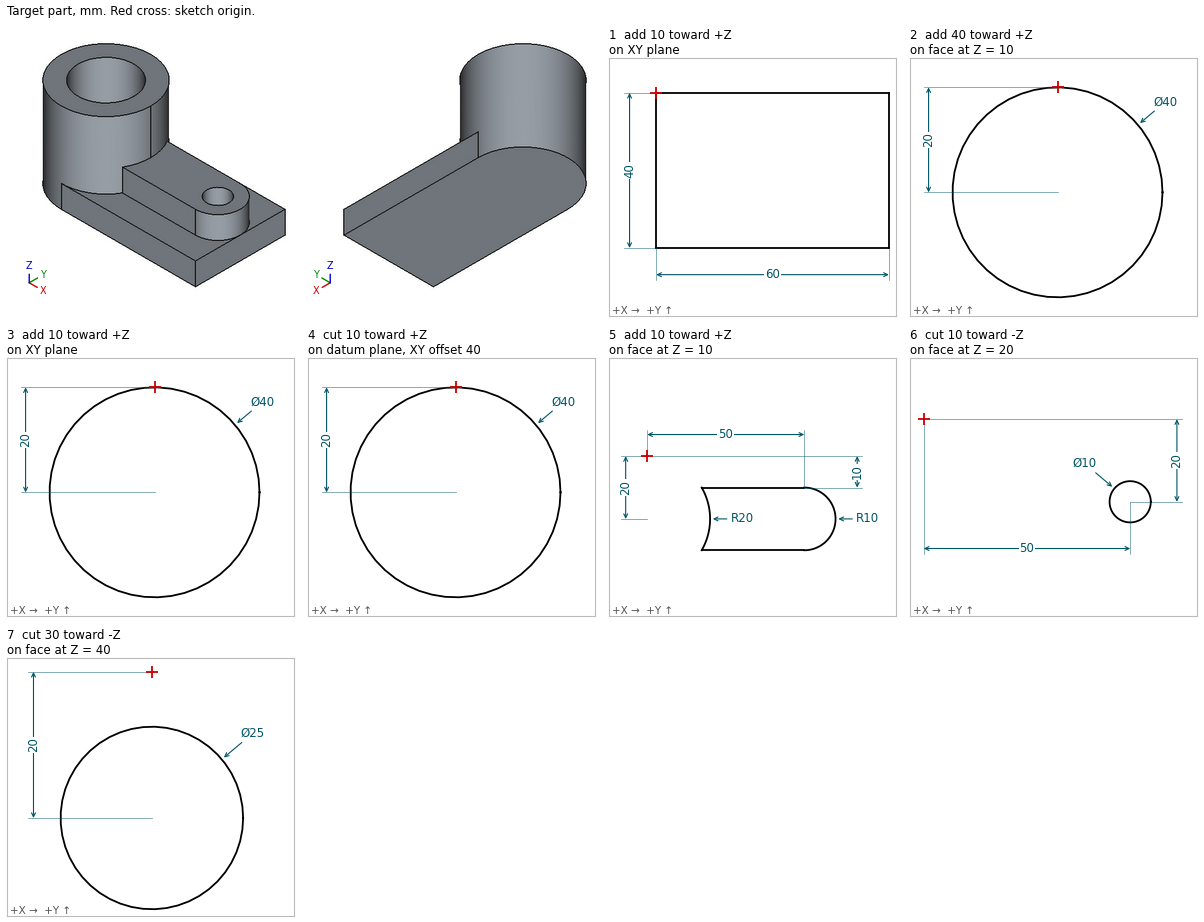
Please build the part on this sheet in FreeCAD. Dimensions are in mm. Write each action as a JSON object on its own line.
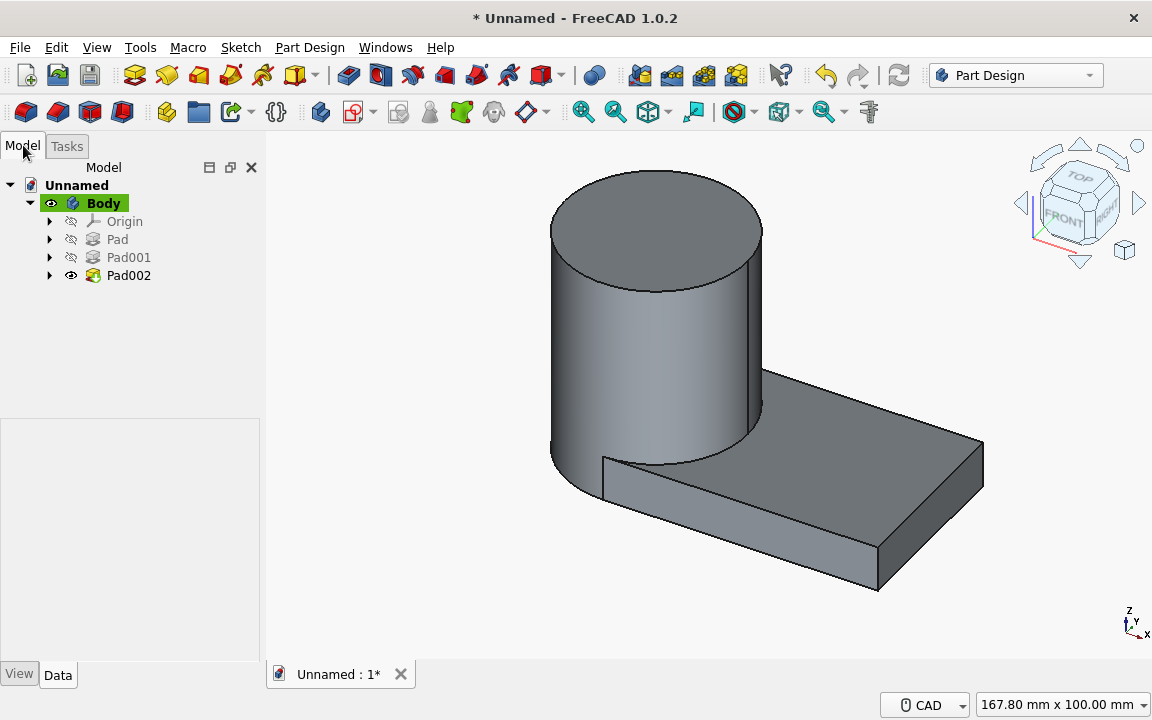
{"action": "left_click", "coordinate": [50, 221]}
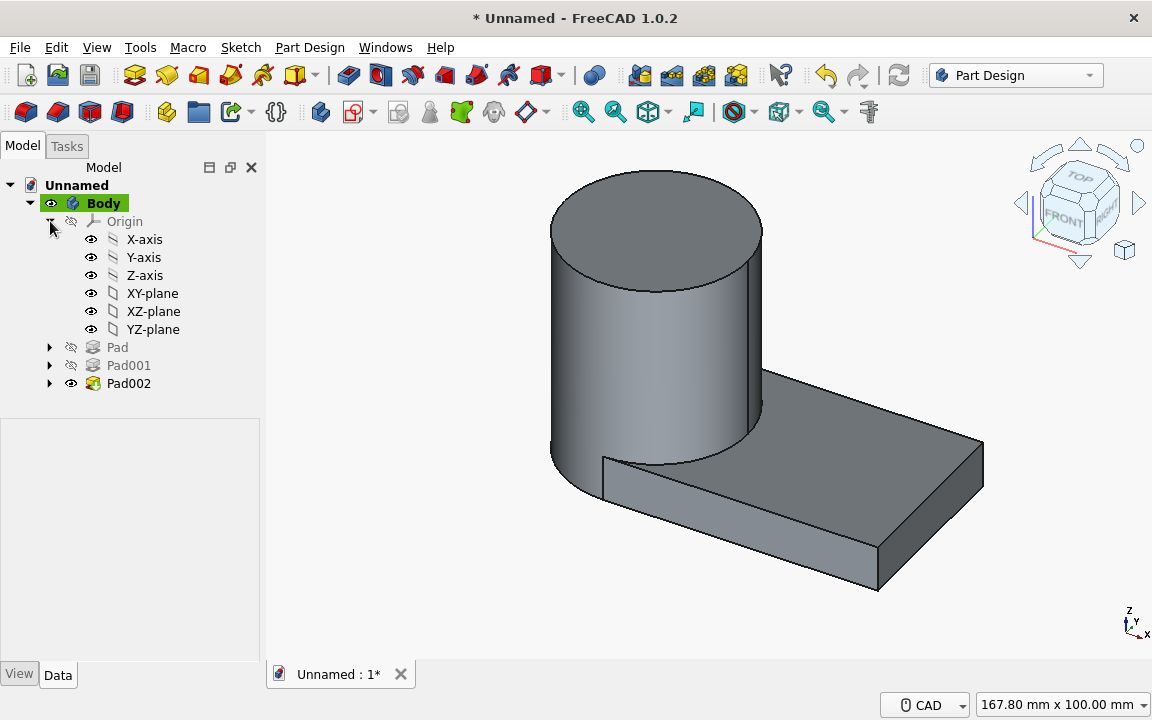
{"action": "left_click", "coordinate": [136, 293]}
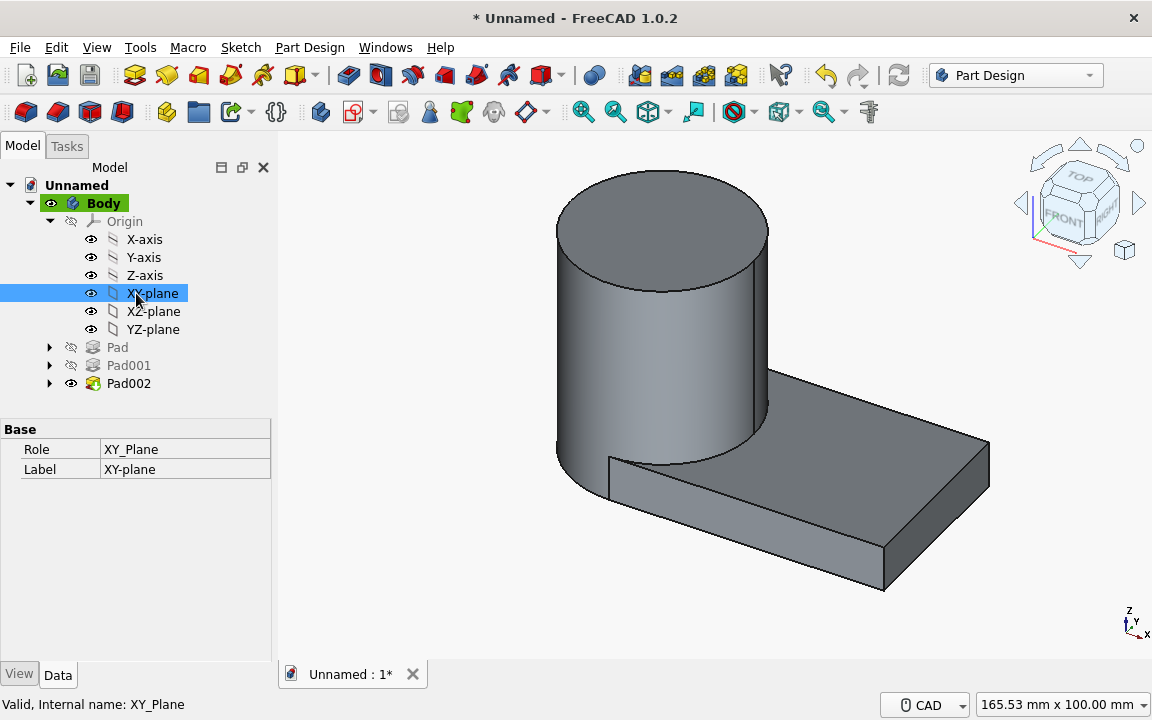
{"action": "left_click", "coordinate": [526, 112]}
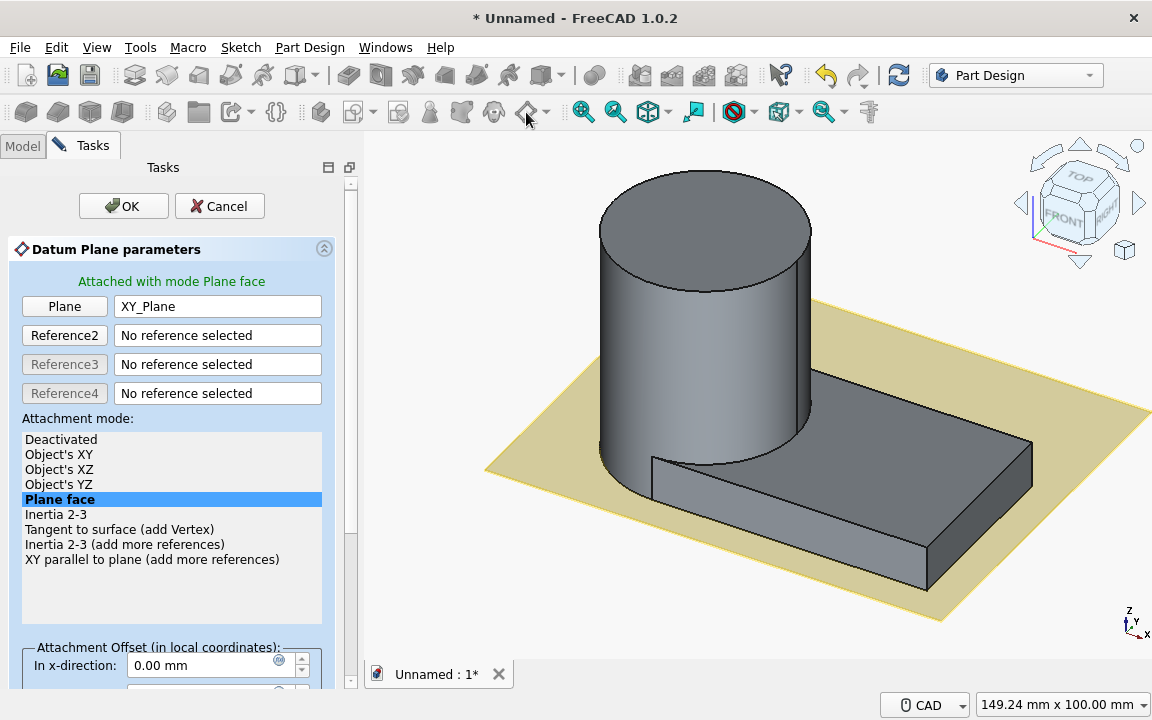
{"action": "scroll", "coordinate": [351, 432], "scroll_direction": "down", "scroll_amount": 2}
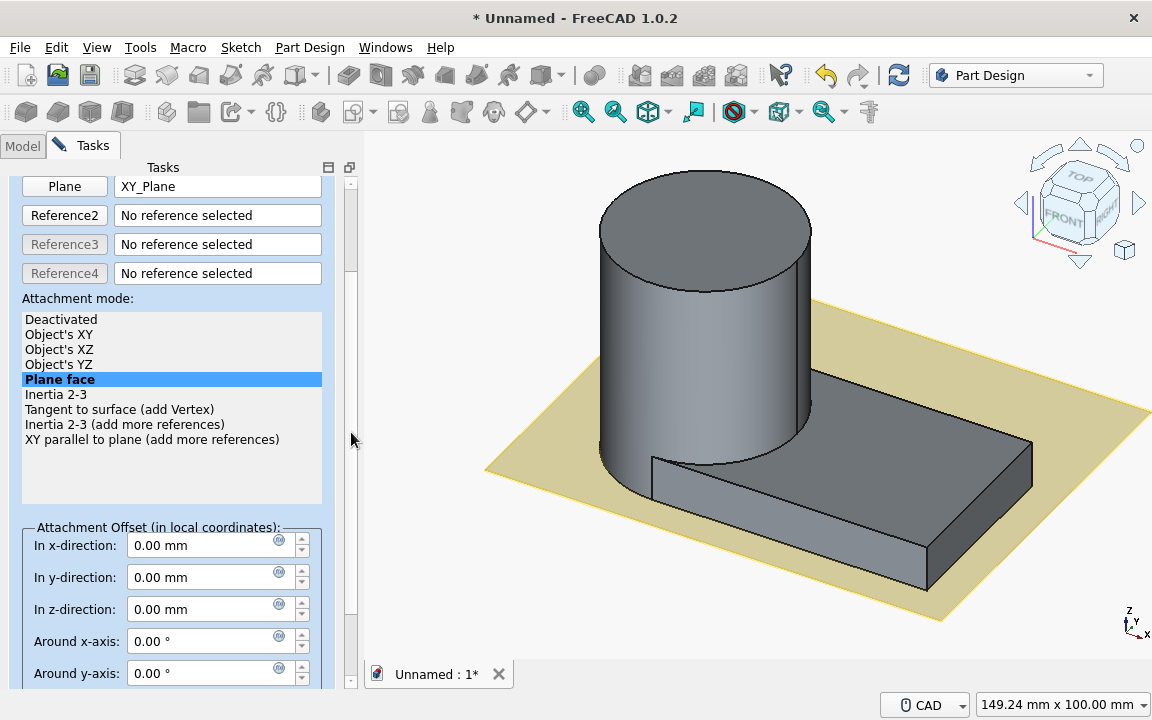
{"action": "triple_click", "coordinate": [210, 609]}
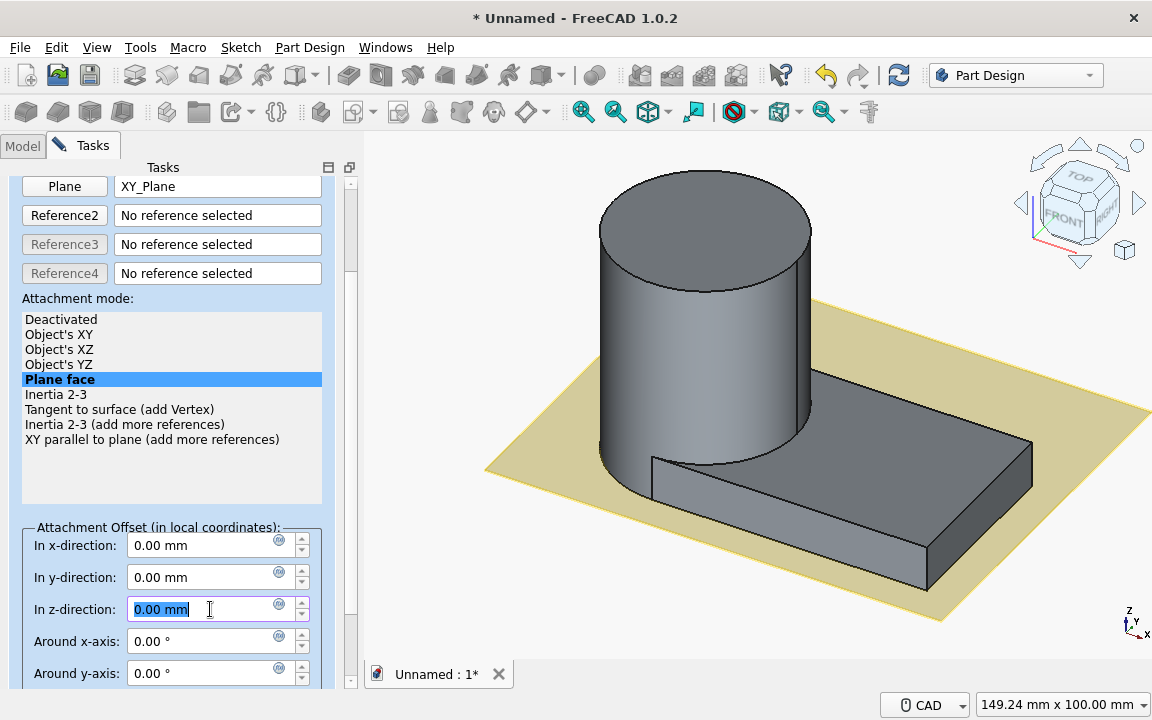
{"action": "type", "text": "40"}
{"action": "key", "text": "Tab"}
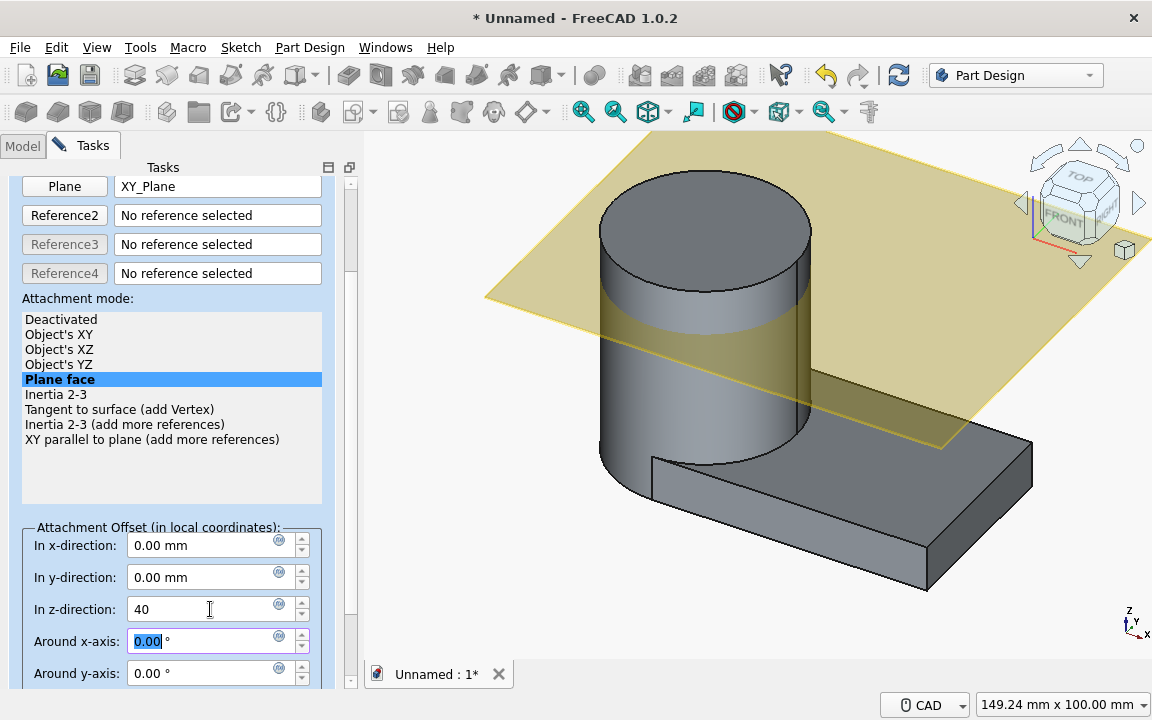
{"action": "scroll", "coordinate": [351, 432], "scroll_direction": "up", "scroll_amount": 3}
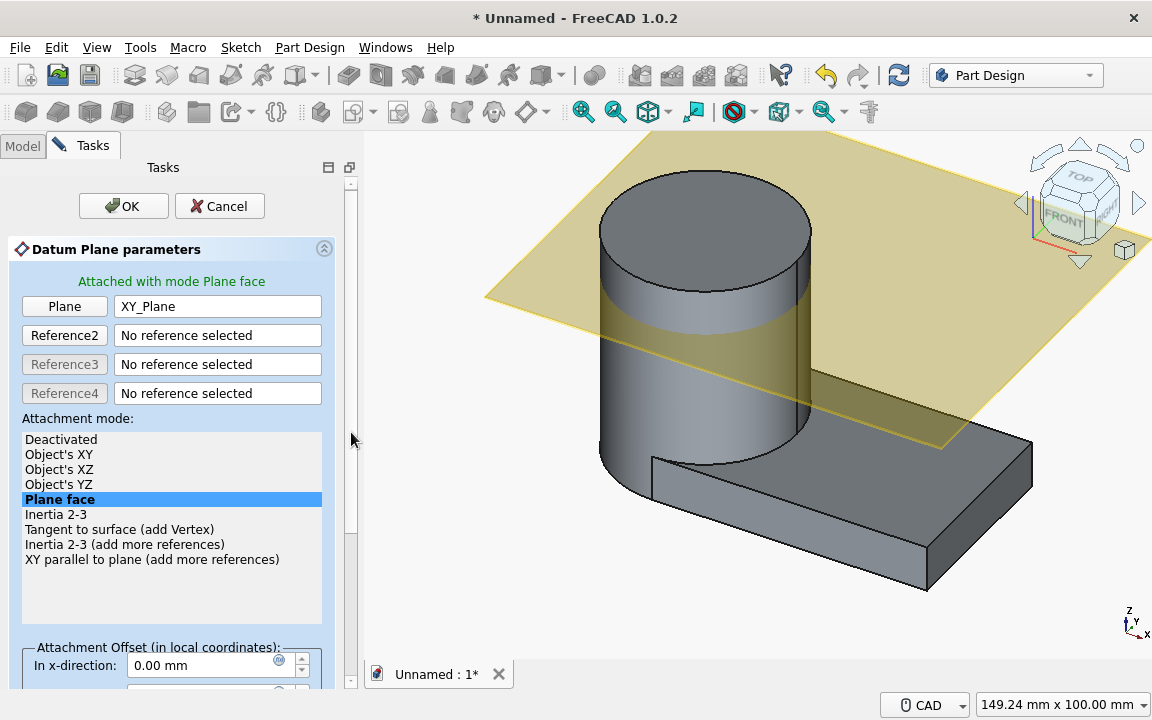
{"action": "left_click", "coordinate": [124, 206]}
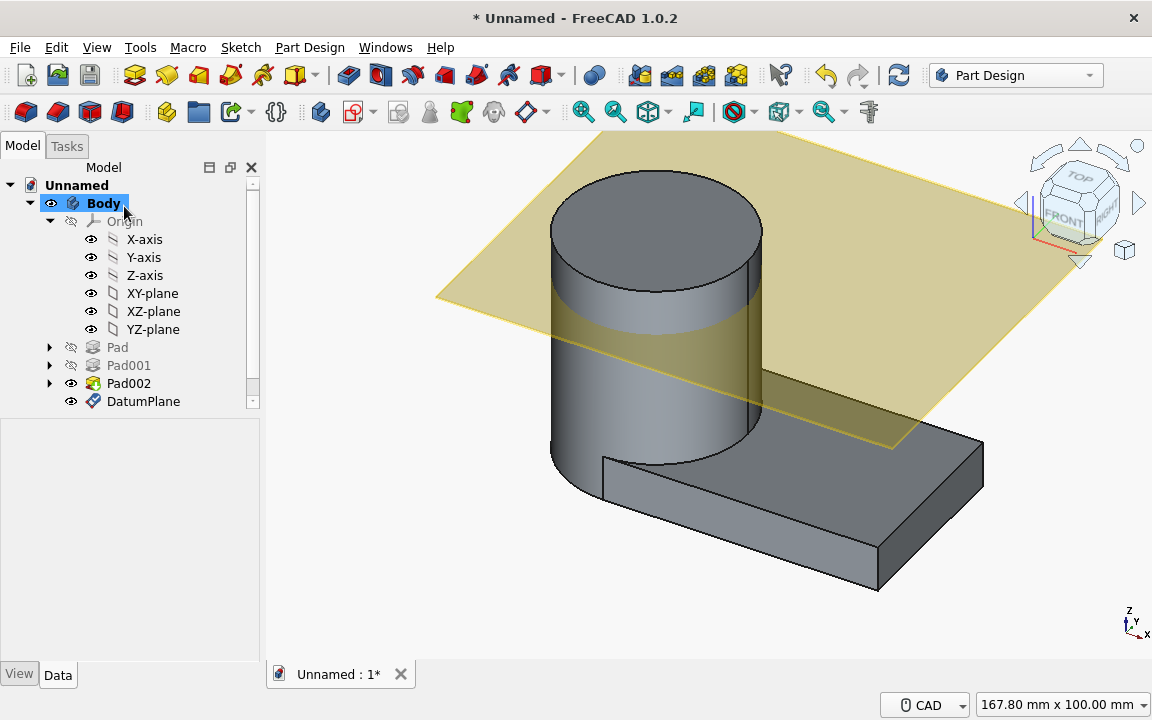
{"action": "left_click", "coordinate": [116, 401]}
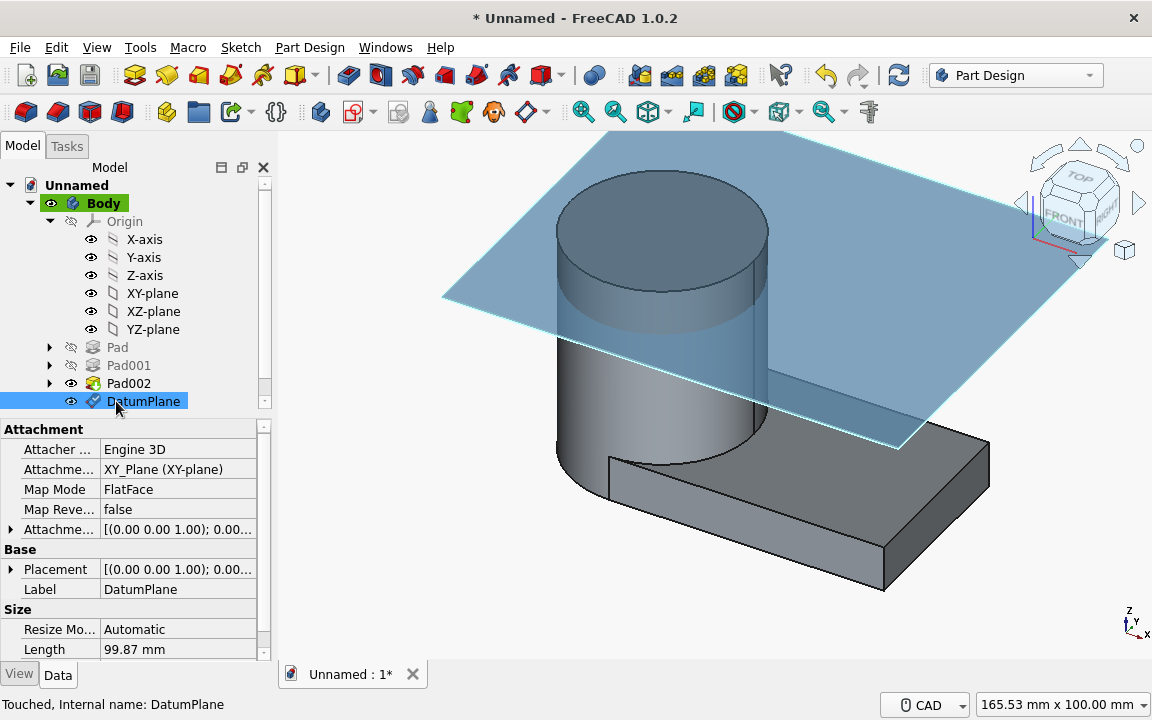
{"action": "left_click", "coordinate": [354, 112]}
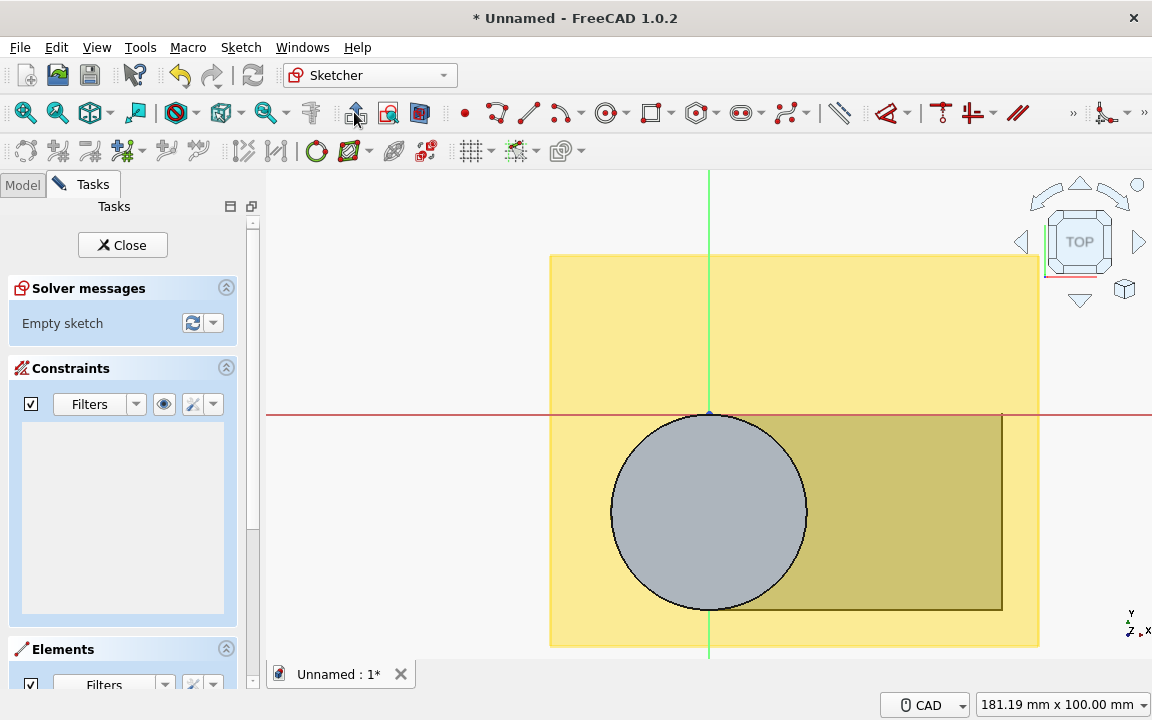
{"action": "left_click", "coordinate": [420, 114]}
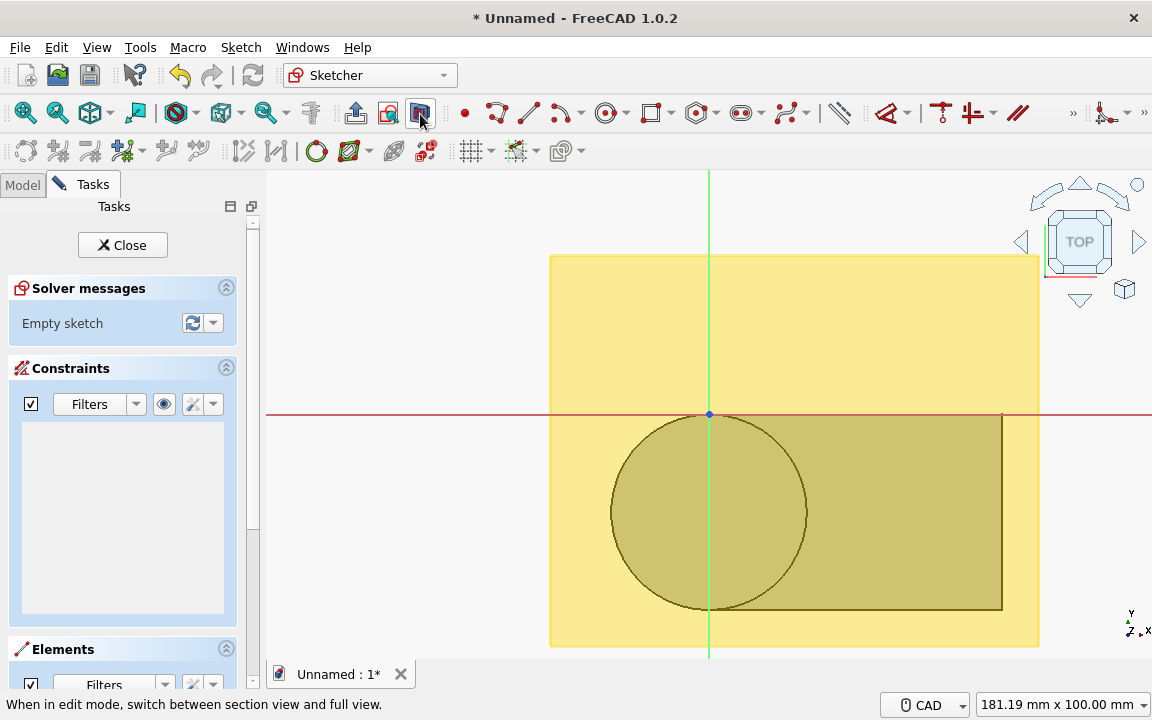
{"action": "scroll", "coordinate": [848, 631], "scroll_direction": "up", "scroll_amount": 2}